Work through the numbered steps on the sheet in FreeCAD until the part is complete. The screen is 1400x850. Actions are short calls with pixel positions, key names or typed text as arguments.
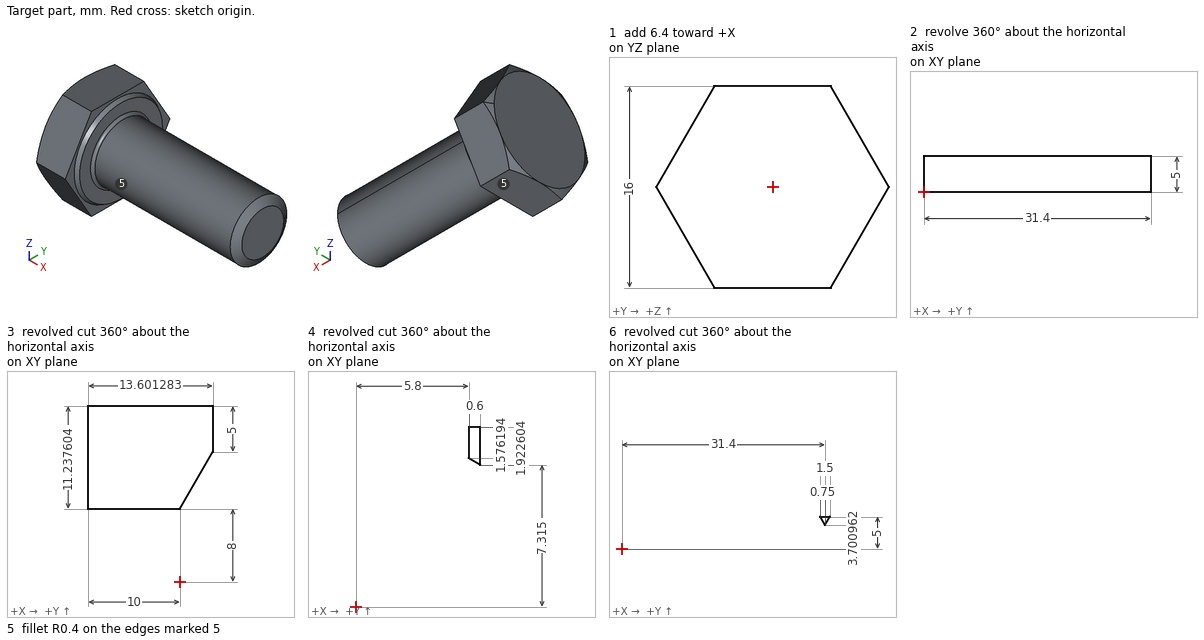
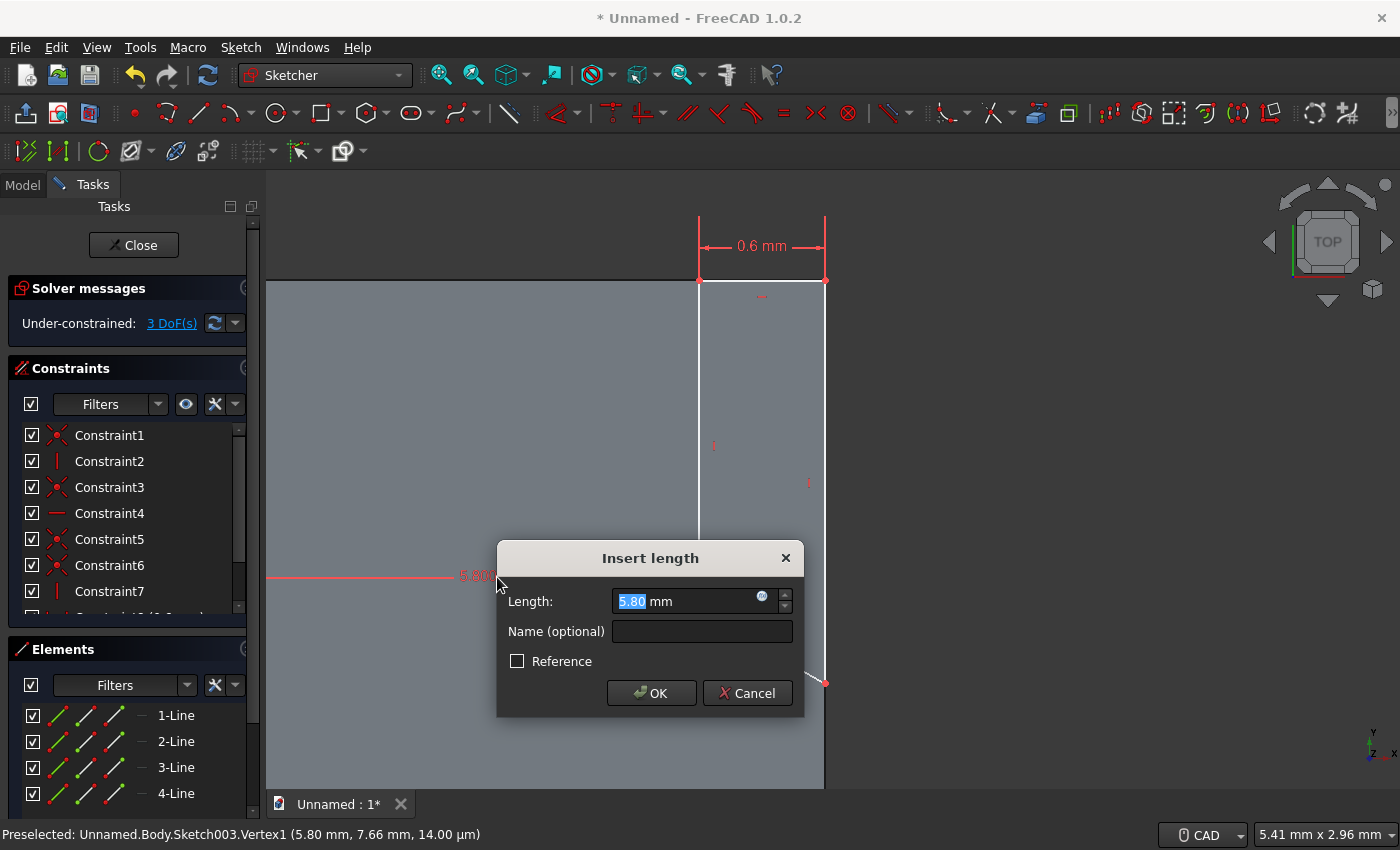
text(5.8)
key(Return)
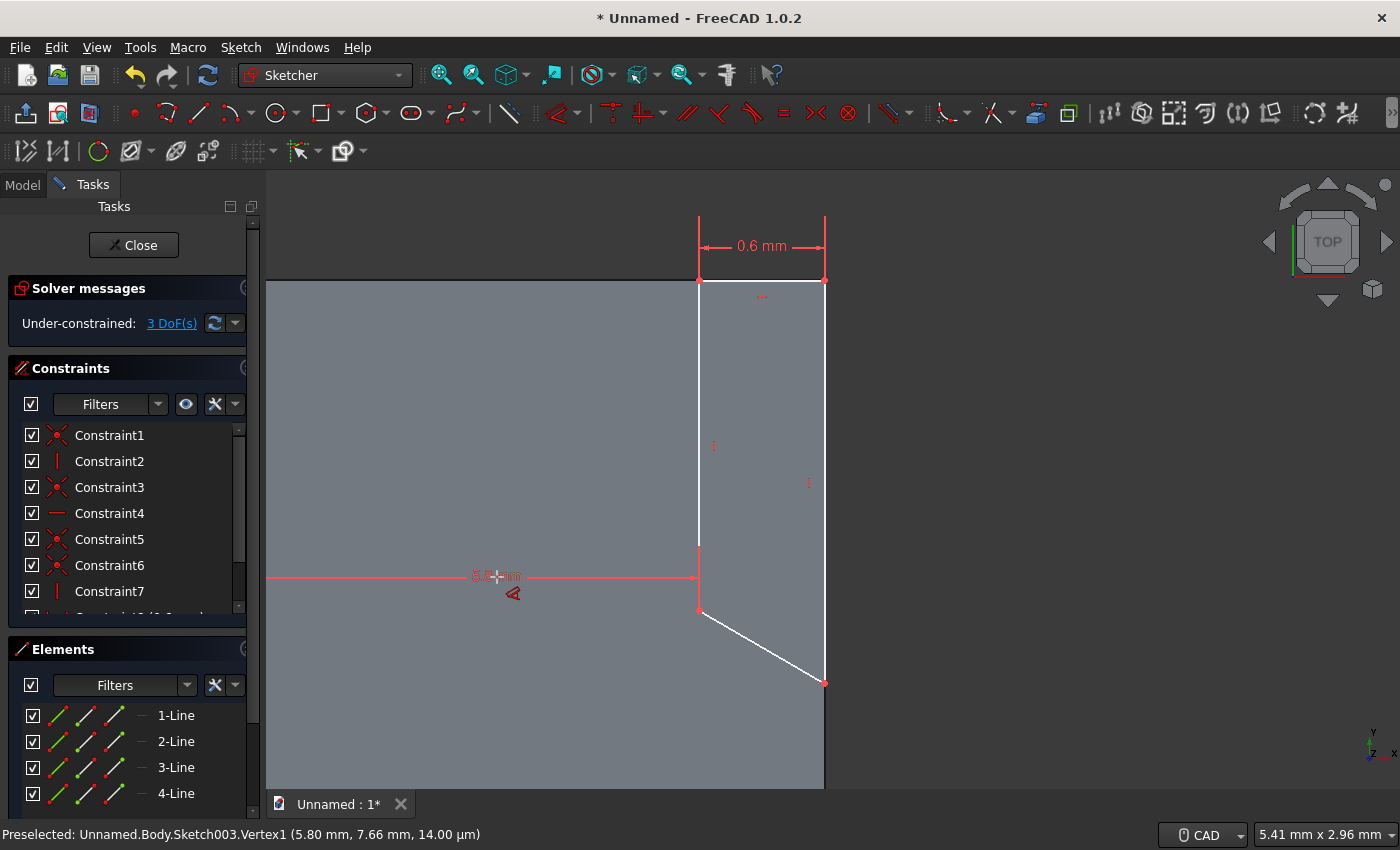
click(825, 684)
click(859, 722)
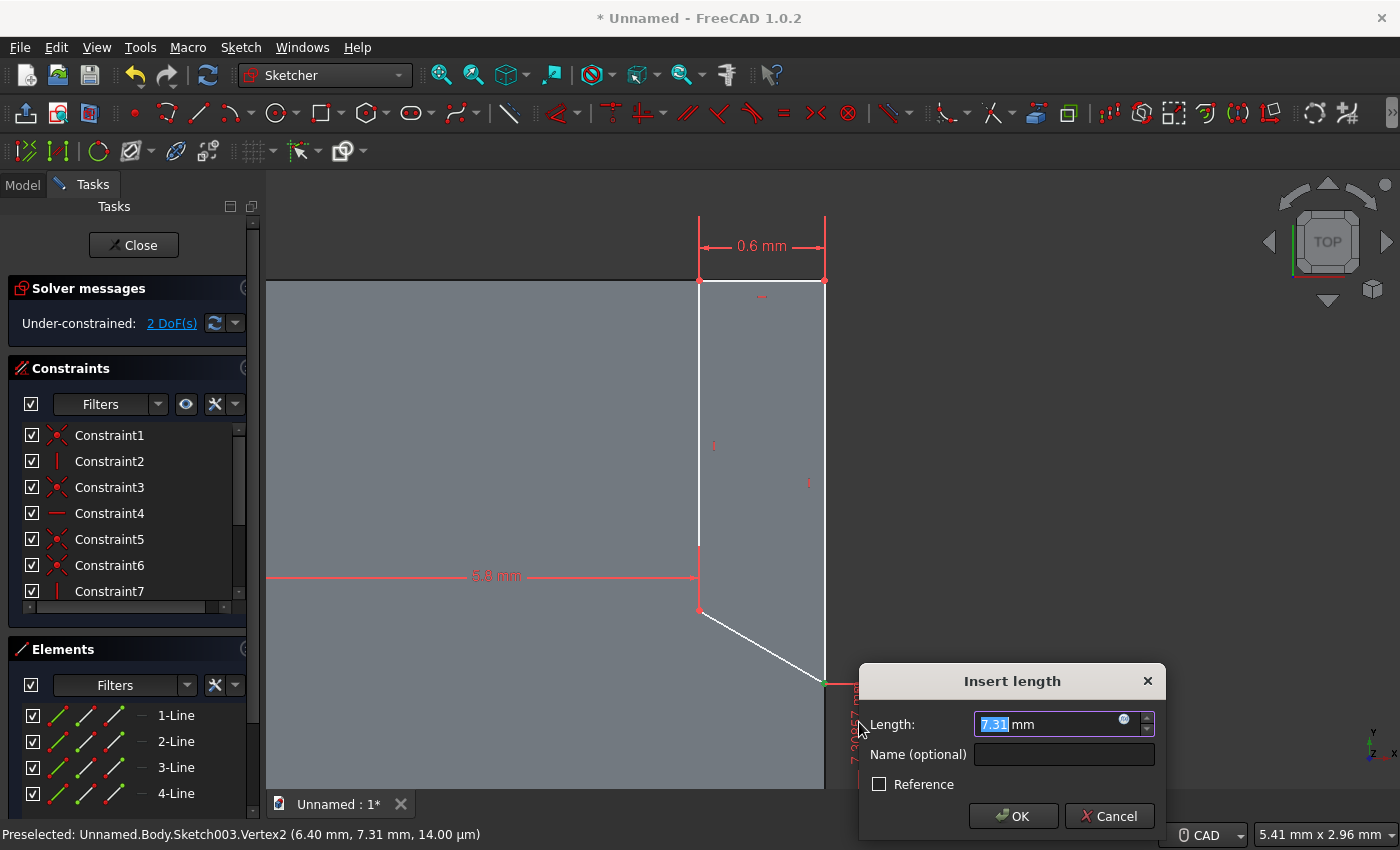
text(7.315)
key(Return)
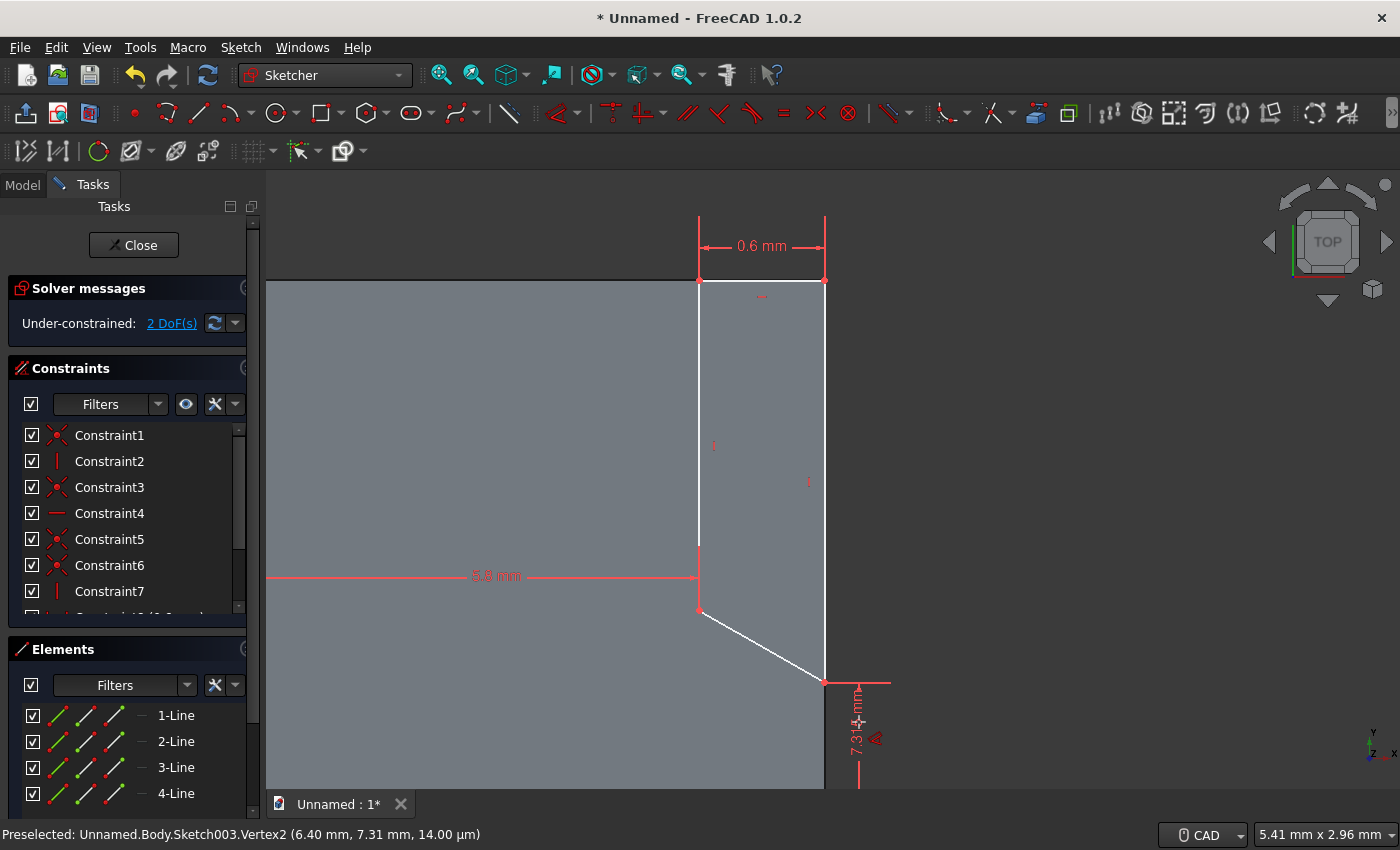
click(825, 562)
click(859, 482)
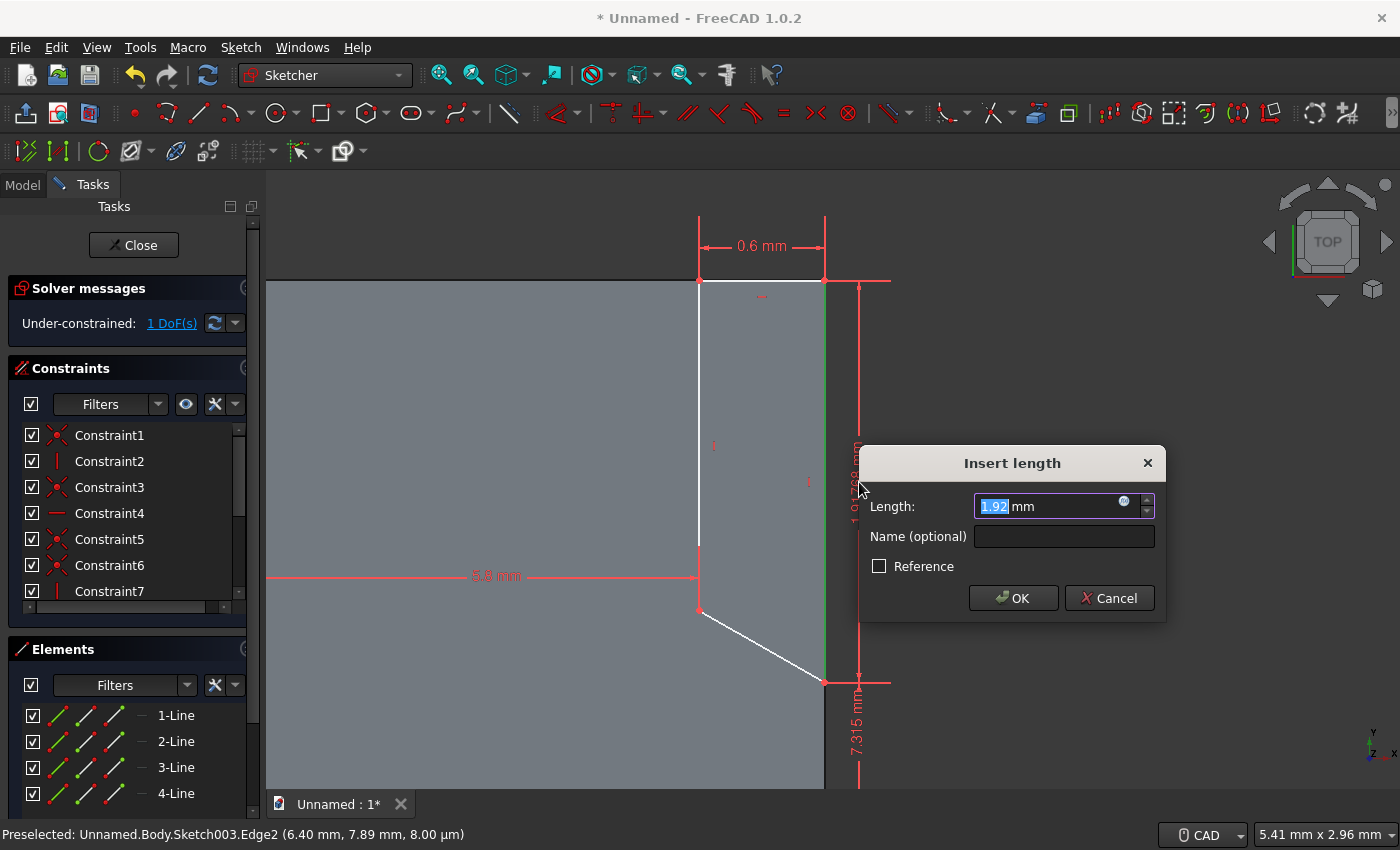
text(1.922604)
key(Return)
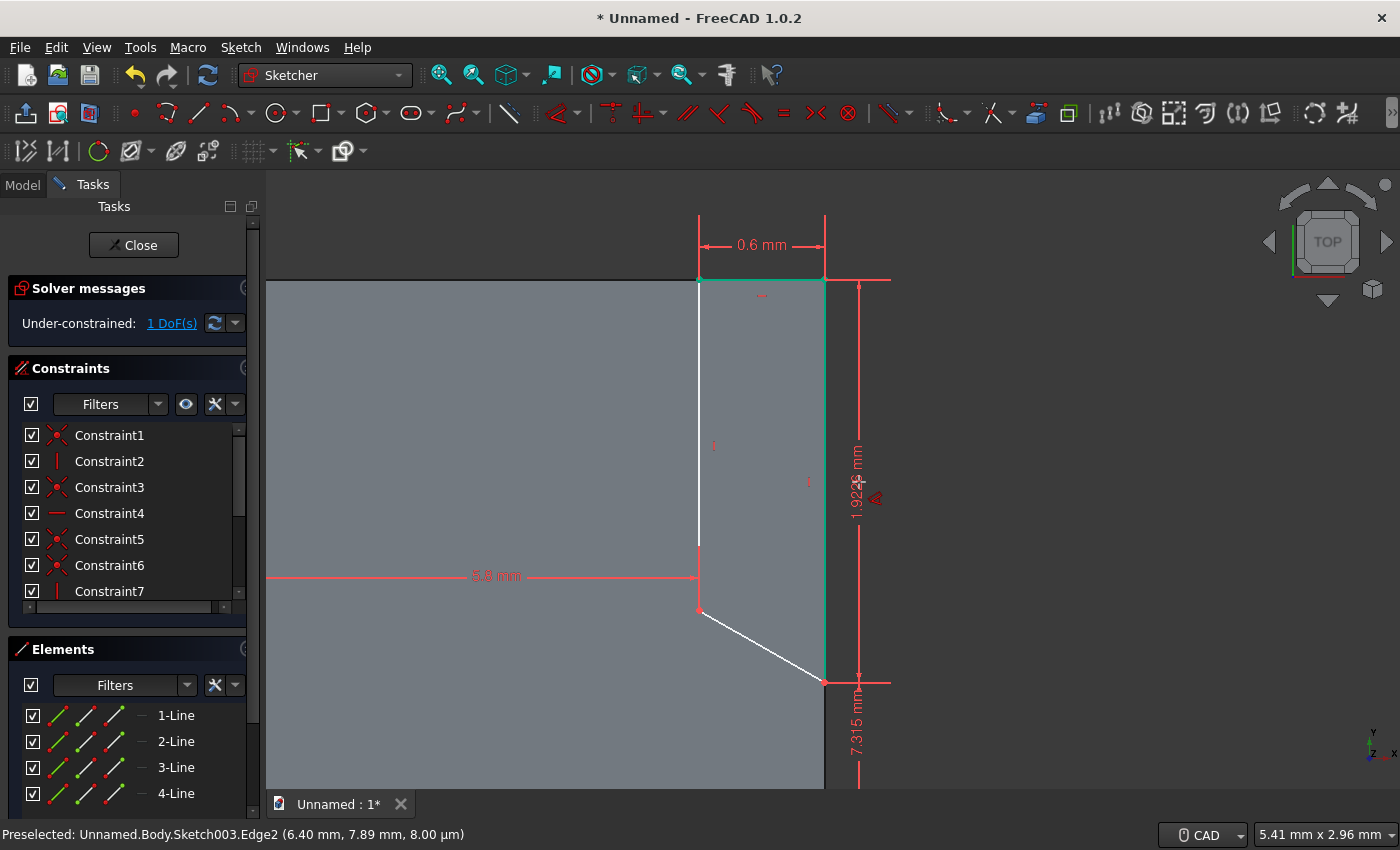
click(699, 379)
click(665, 445)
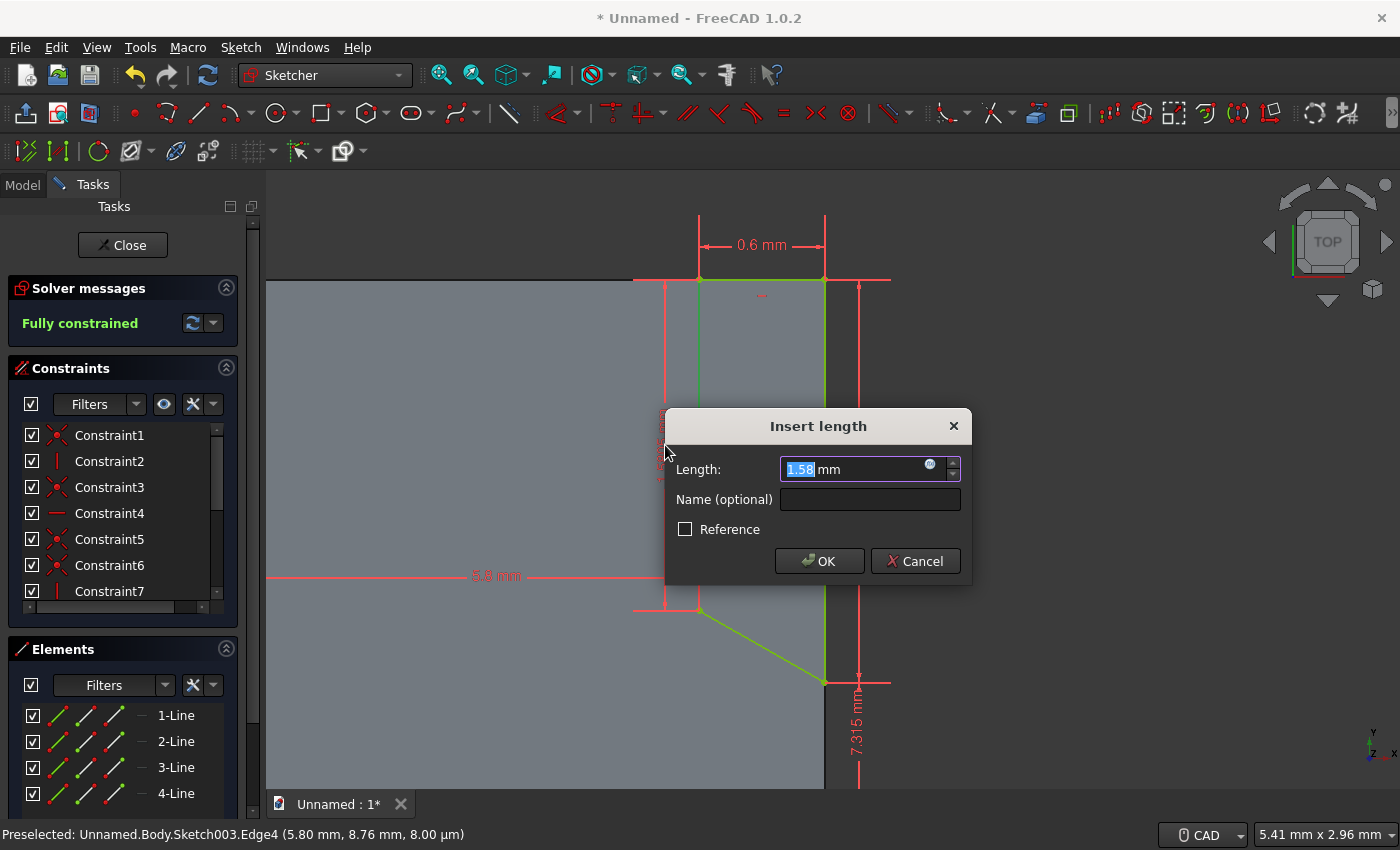
text(1.576194)
key(Return)
key(Escape)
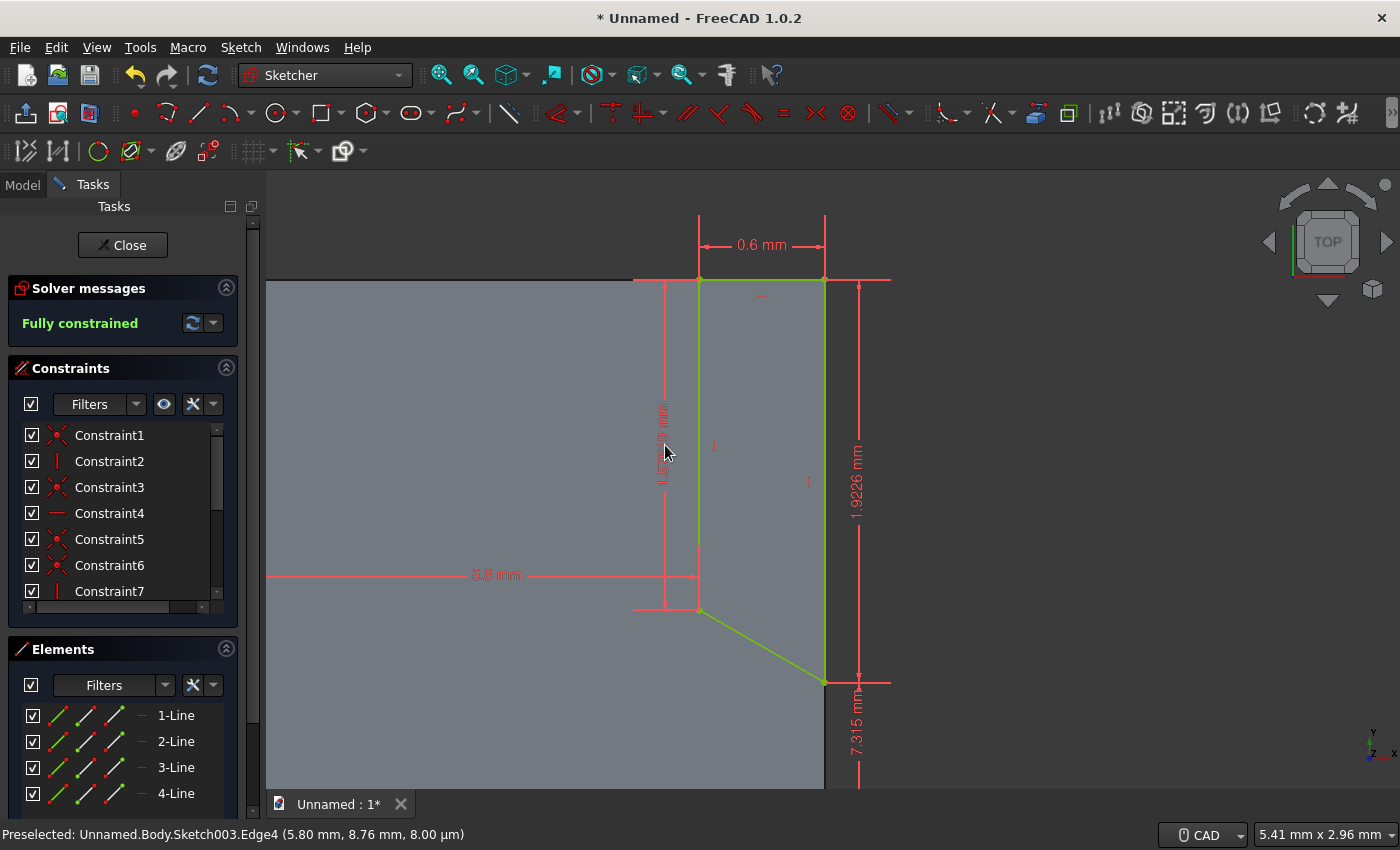
click(123, 245)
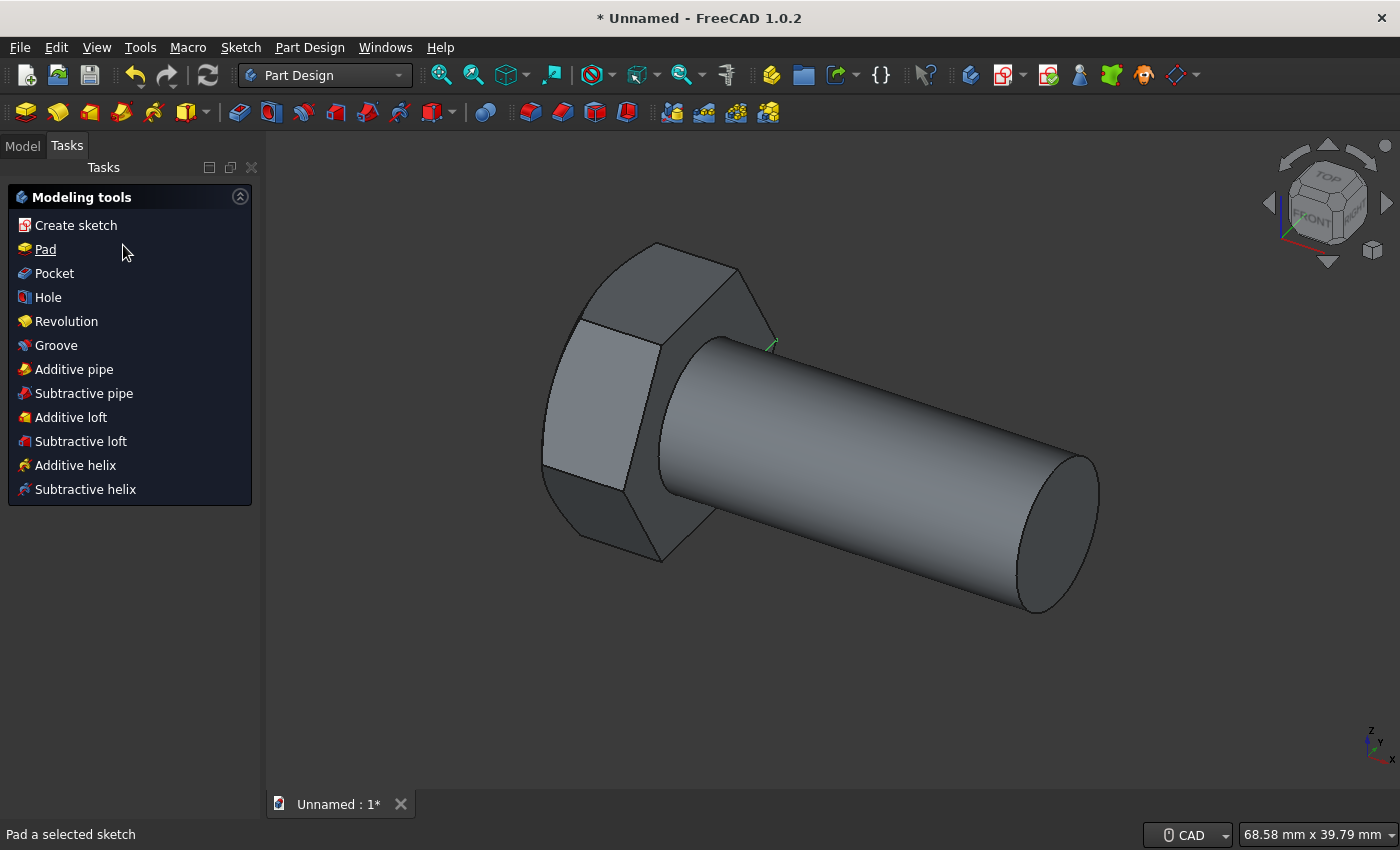
click(304, 112)